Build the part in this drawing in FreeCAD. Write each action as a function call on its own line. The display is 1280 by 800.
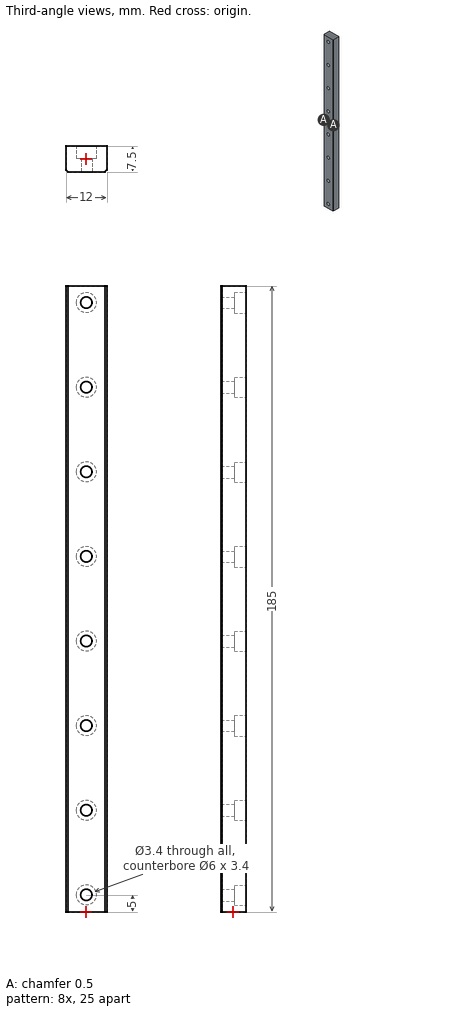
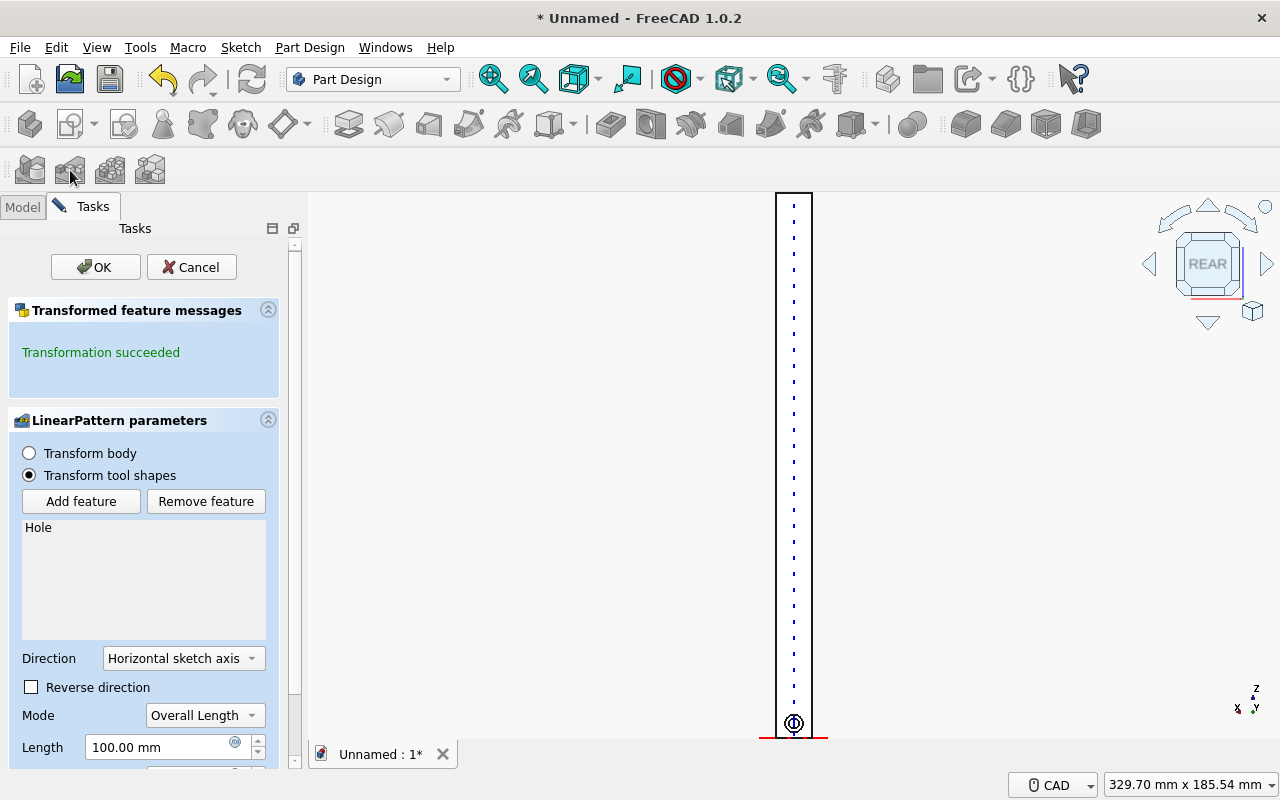
click(184, 658)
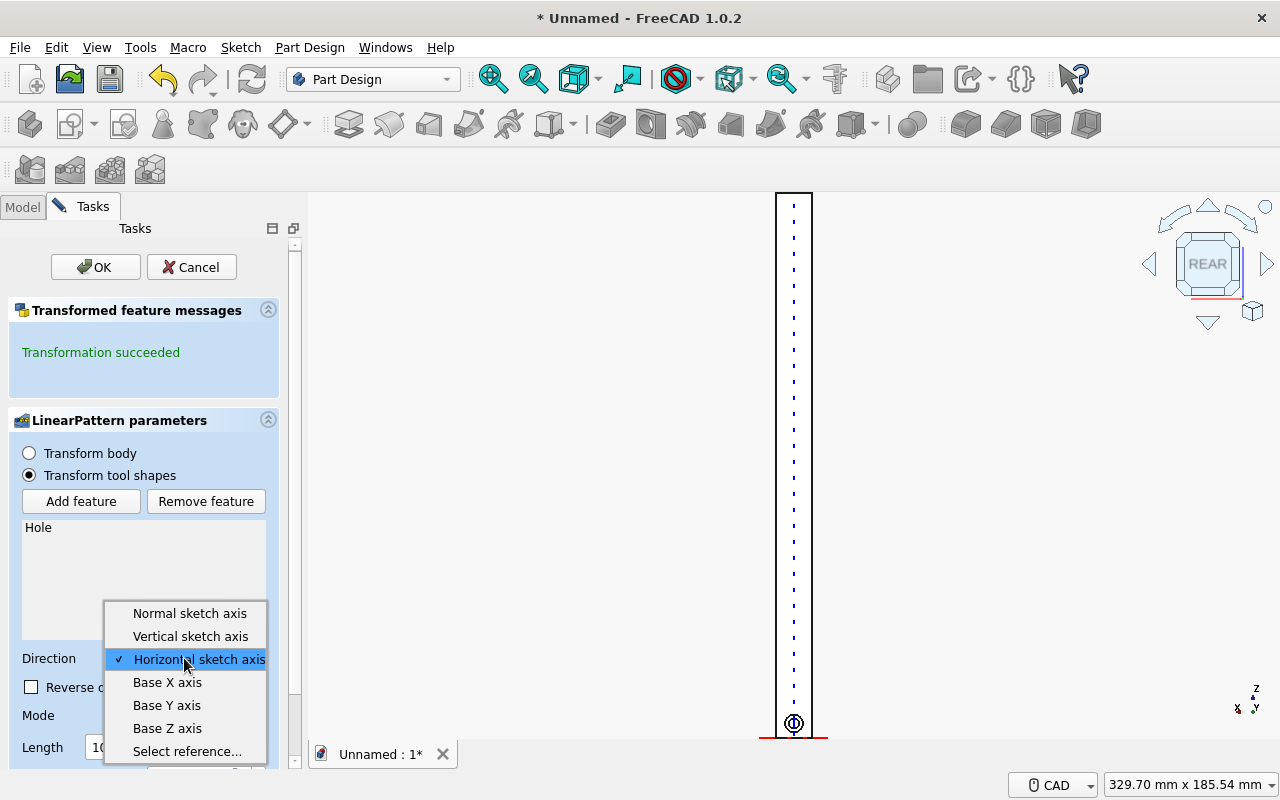
click(184, 728)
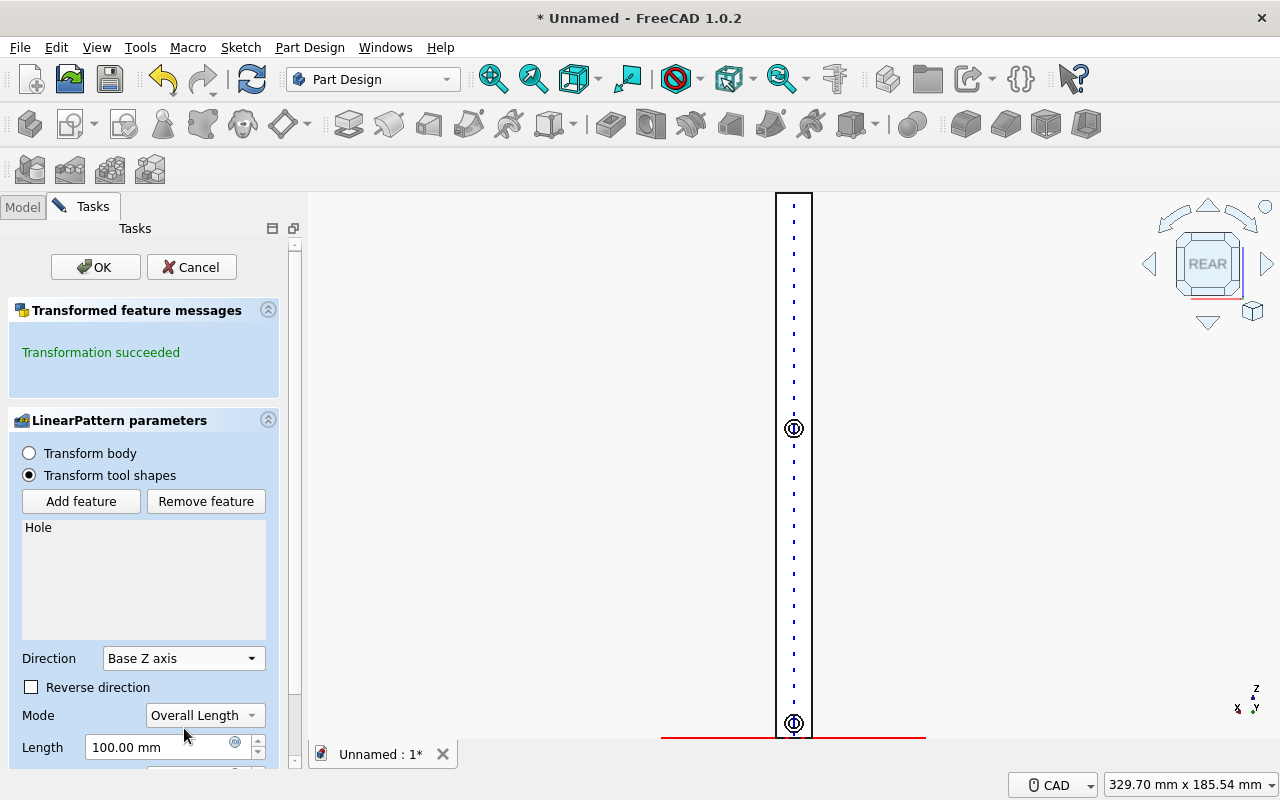
click(206, 716)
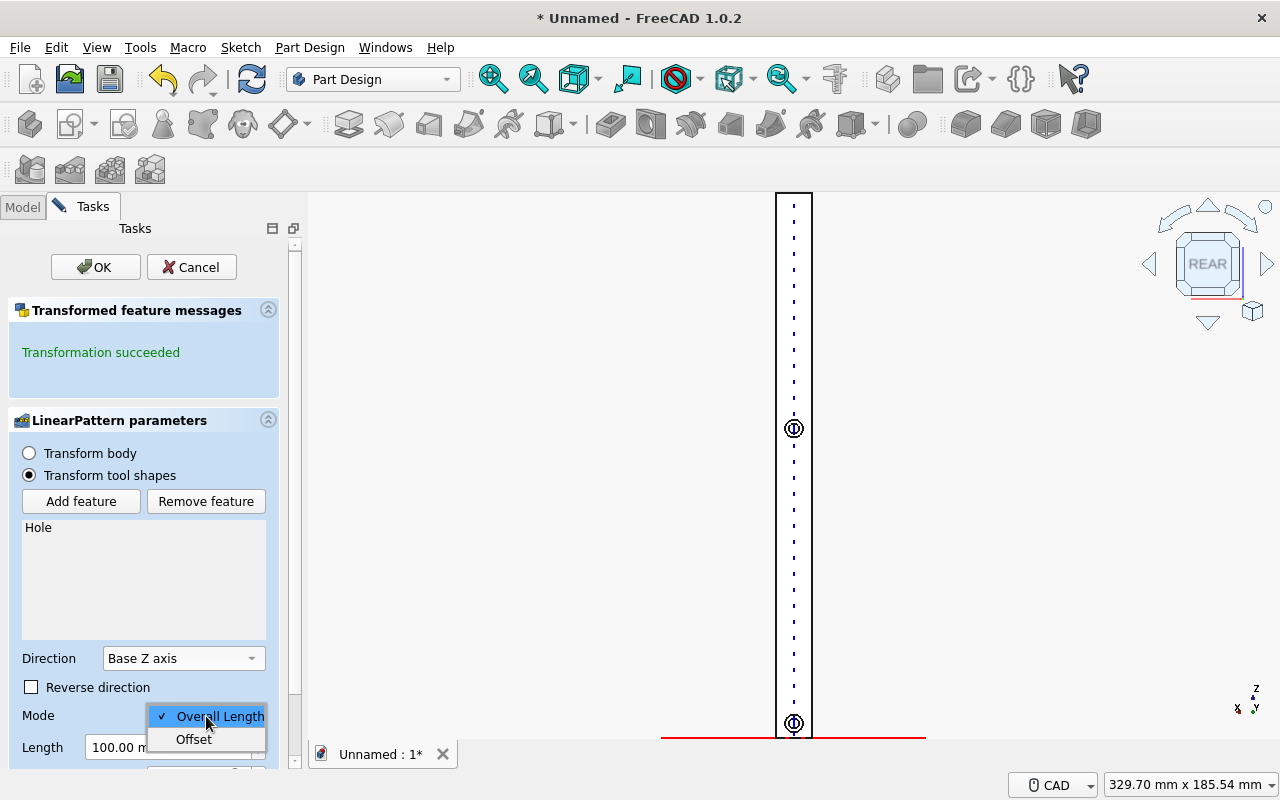
click(206, 740)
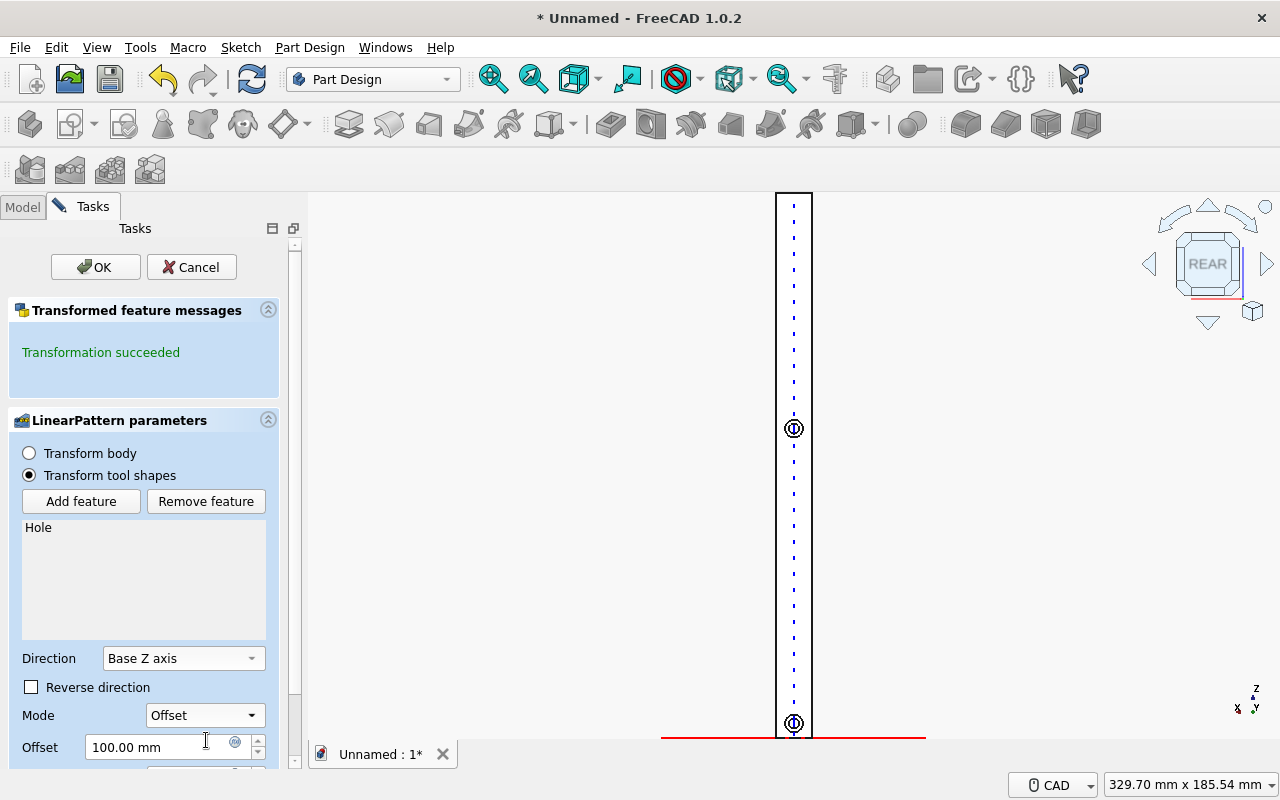
triple_click(168, 747)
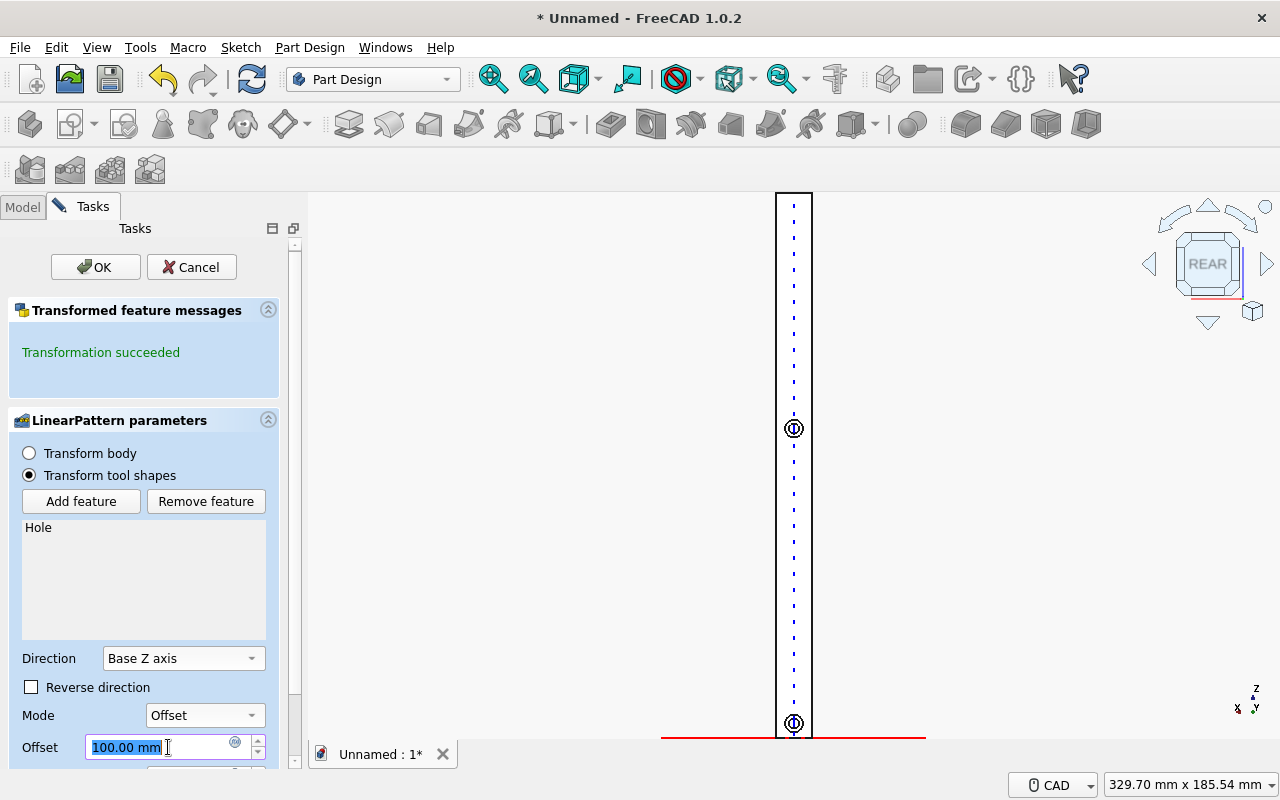
text(25)
key(Tab)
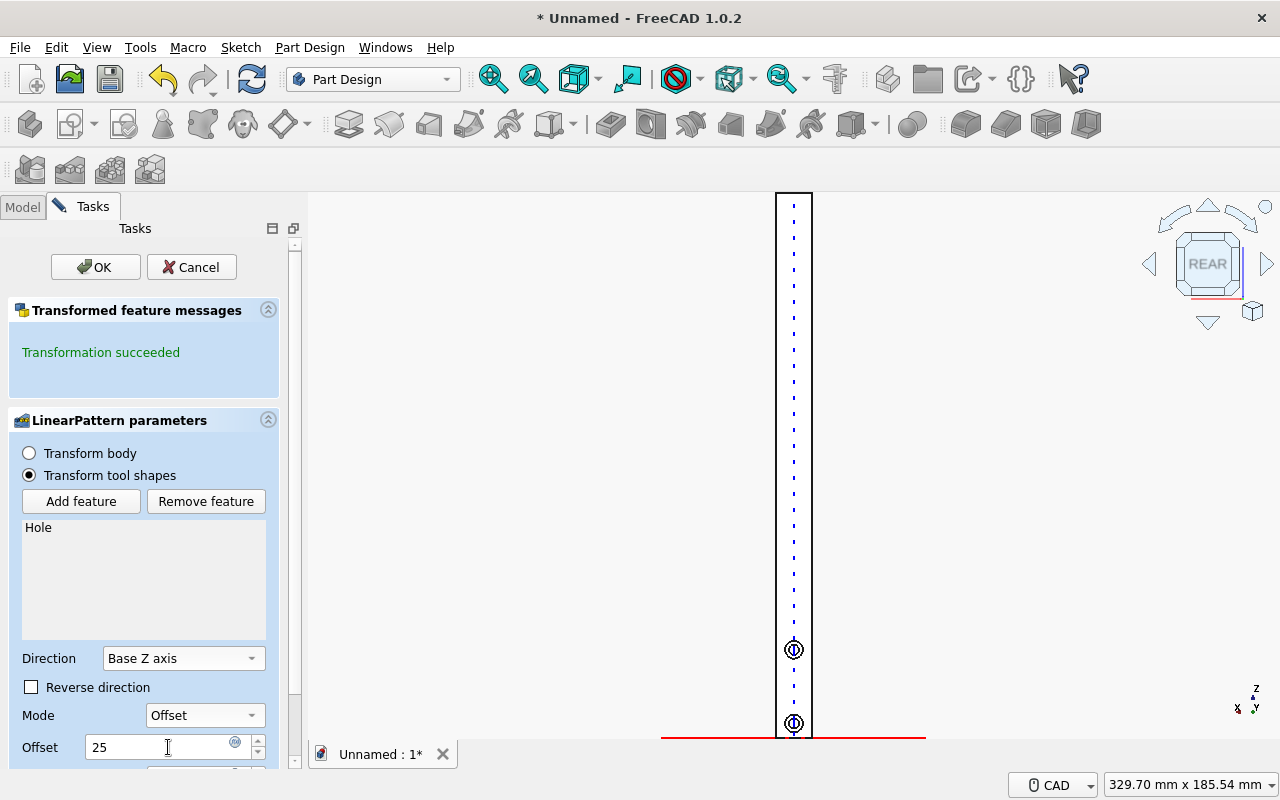
scroll(295, 503, down, 2)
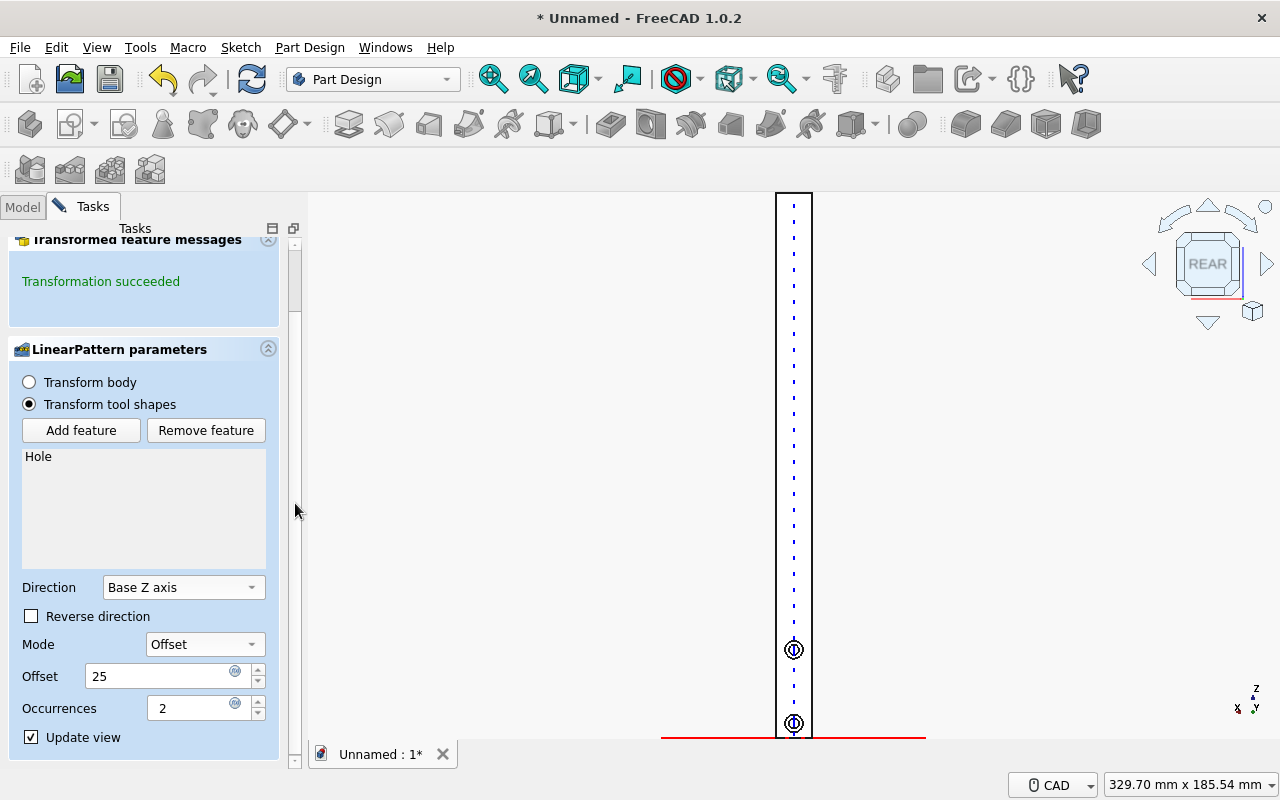
triple_click(198, 708)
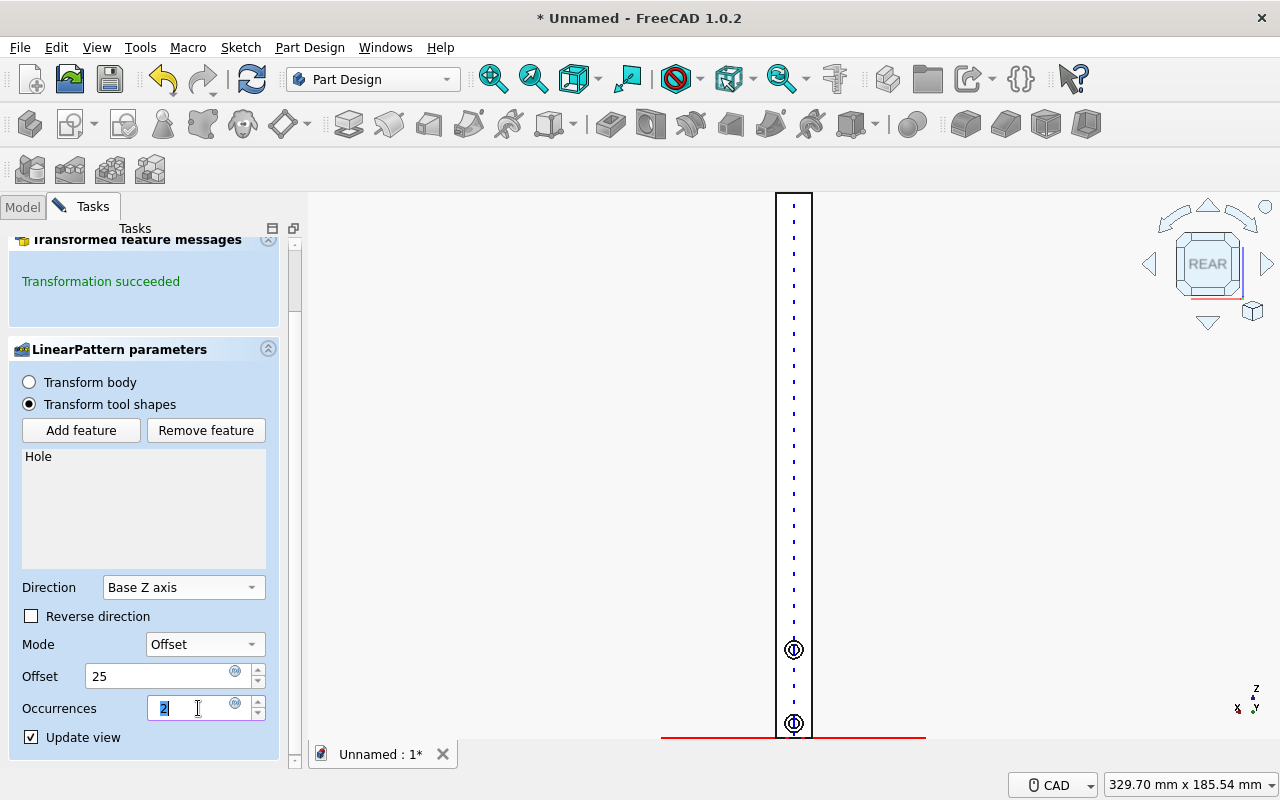
text(8)
key(Tab)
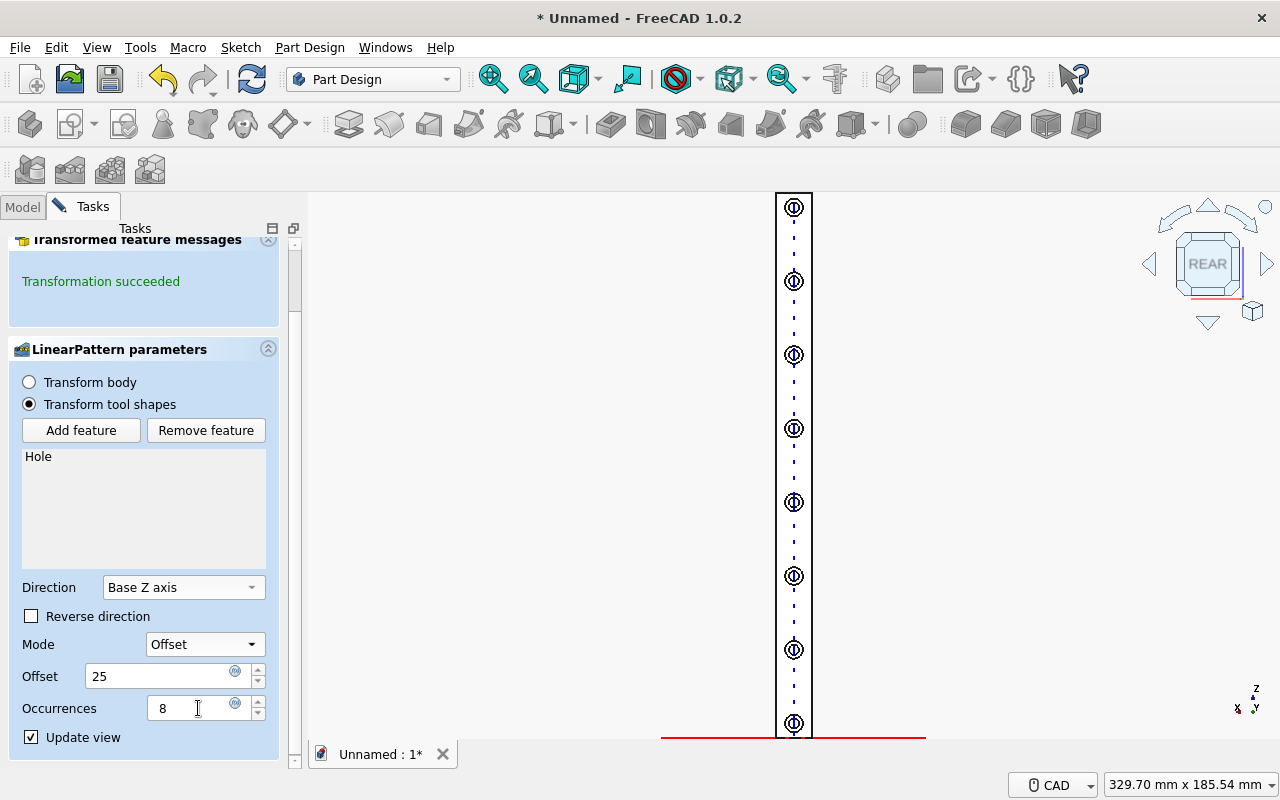
scroll(295, 503, up, 2)